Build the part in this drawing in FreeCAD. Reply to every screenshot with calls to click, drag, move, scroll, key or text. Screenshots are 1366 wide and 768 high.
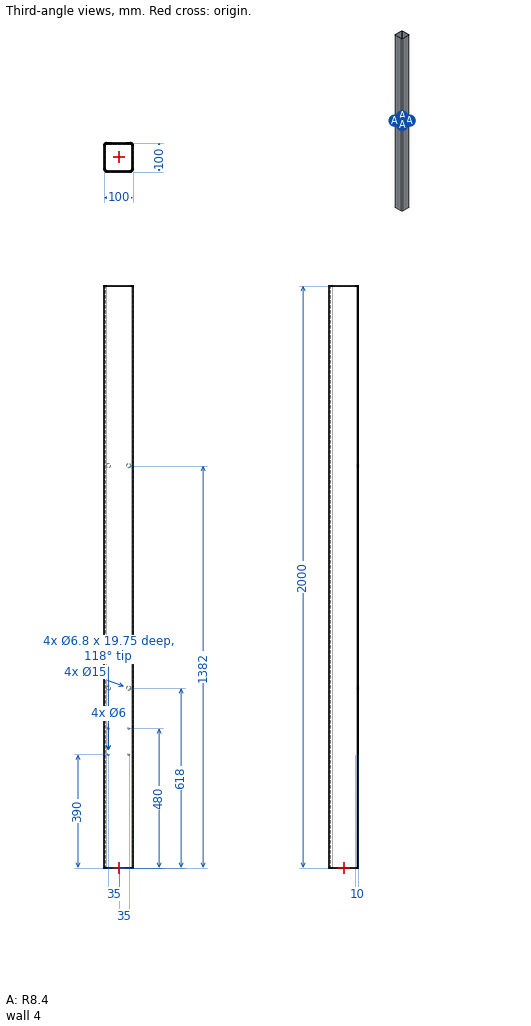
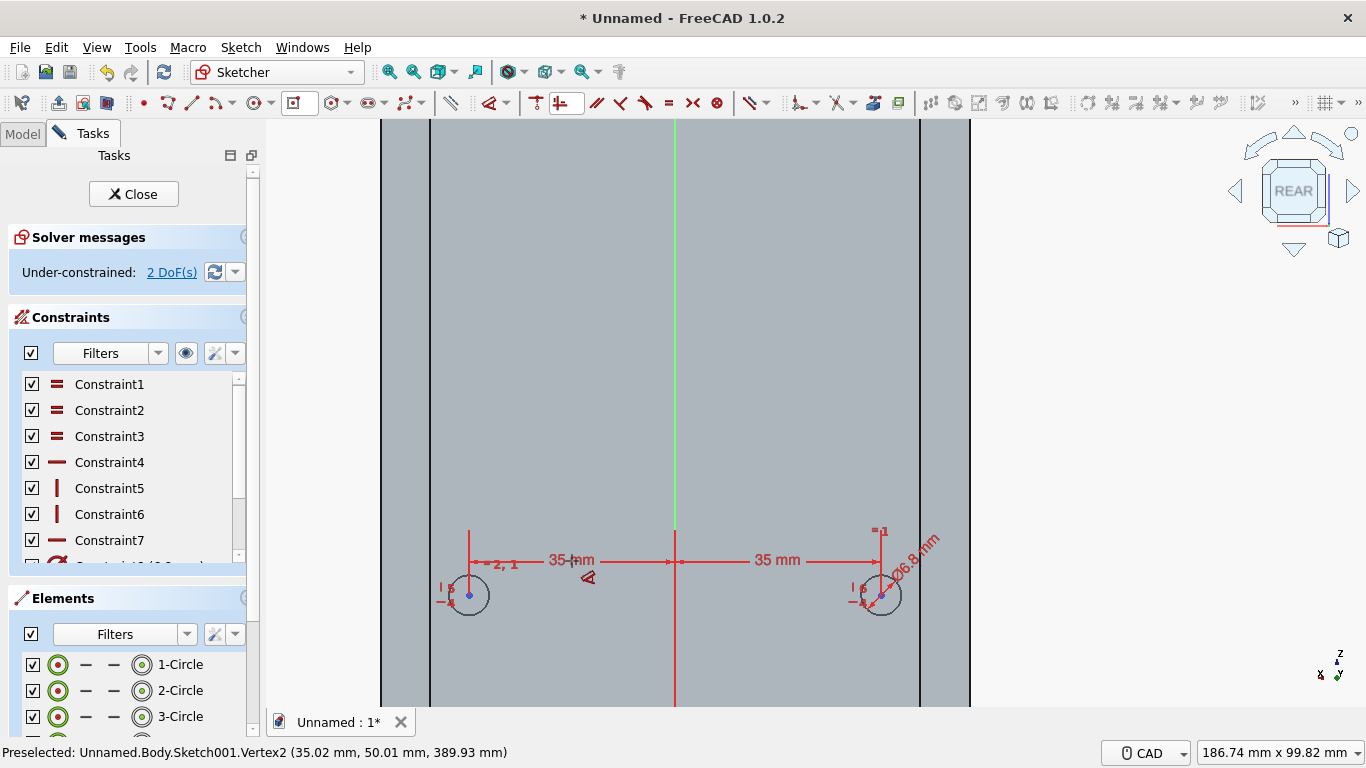
click(881, 595)
click(915, 637)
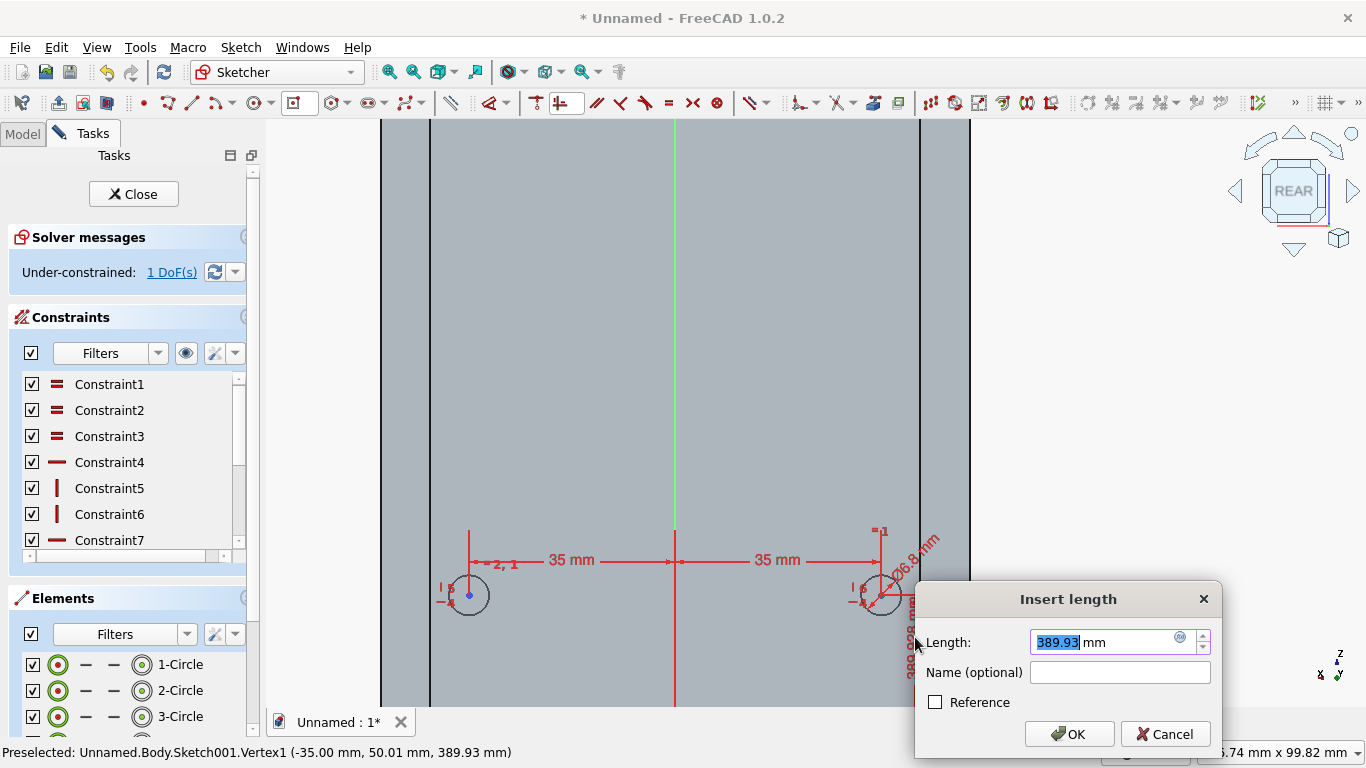
text(390)
key(Return)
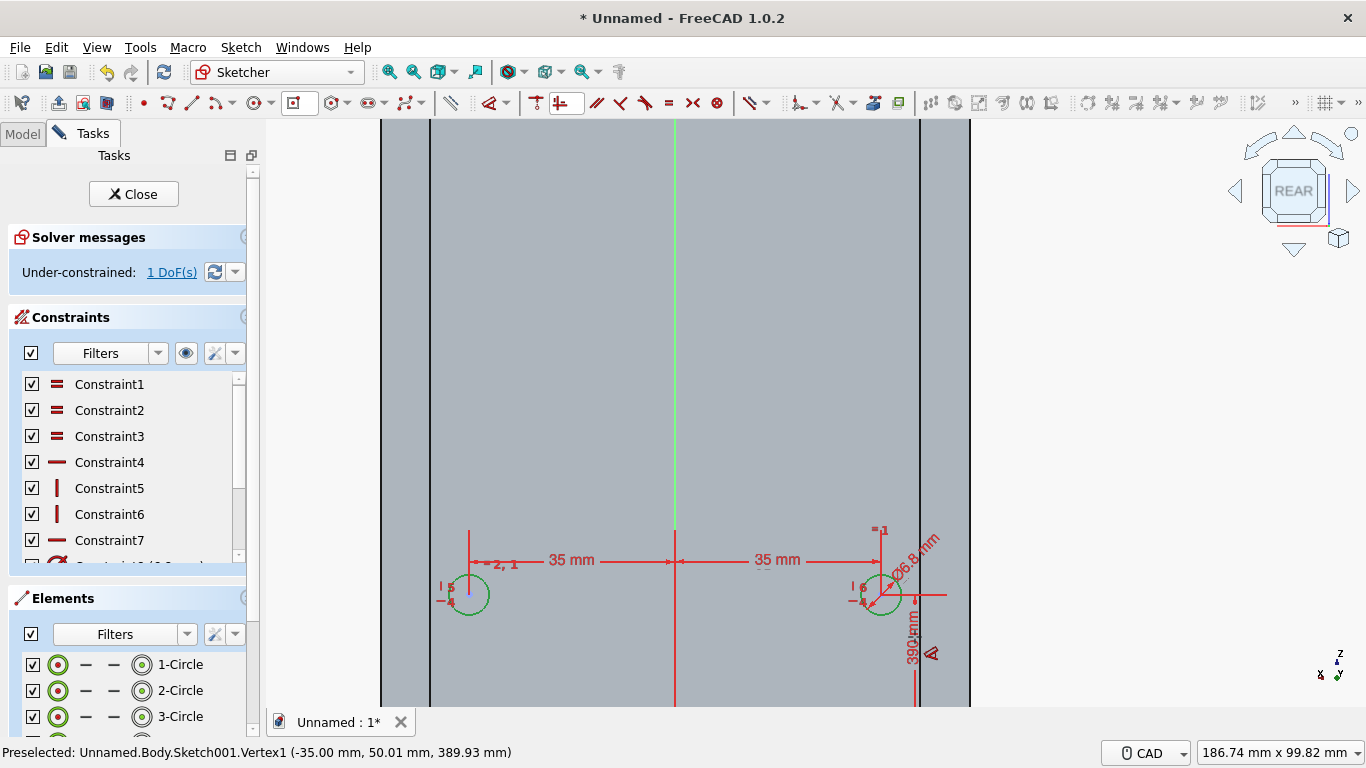
scroll(895, 582, down, 2)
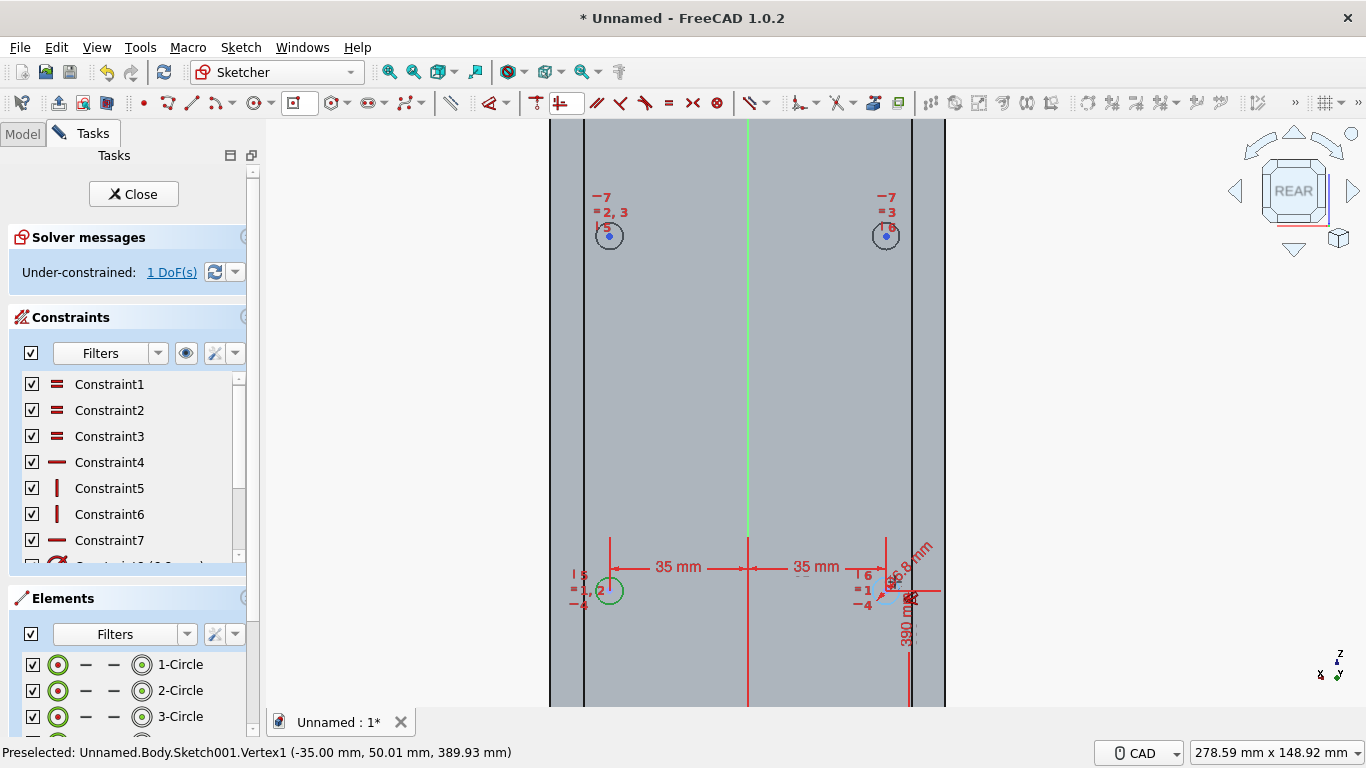
click(610, 236)
click(576, 458)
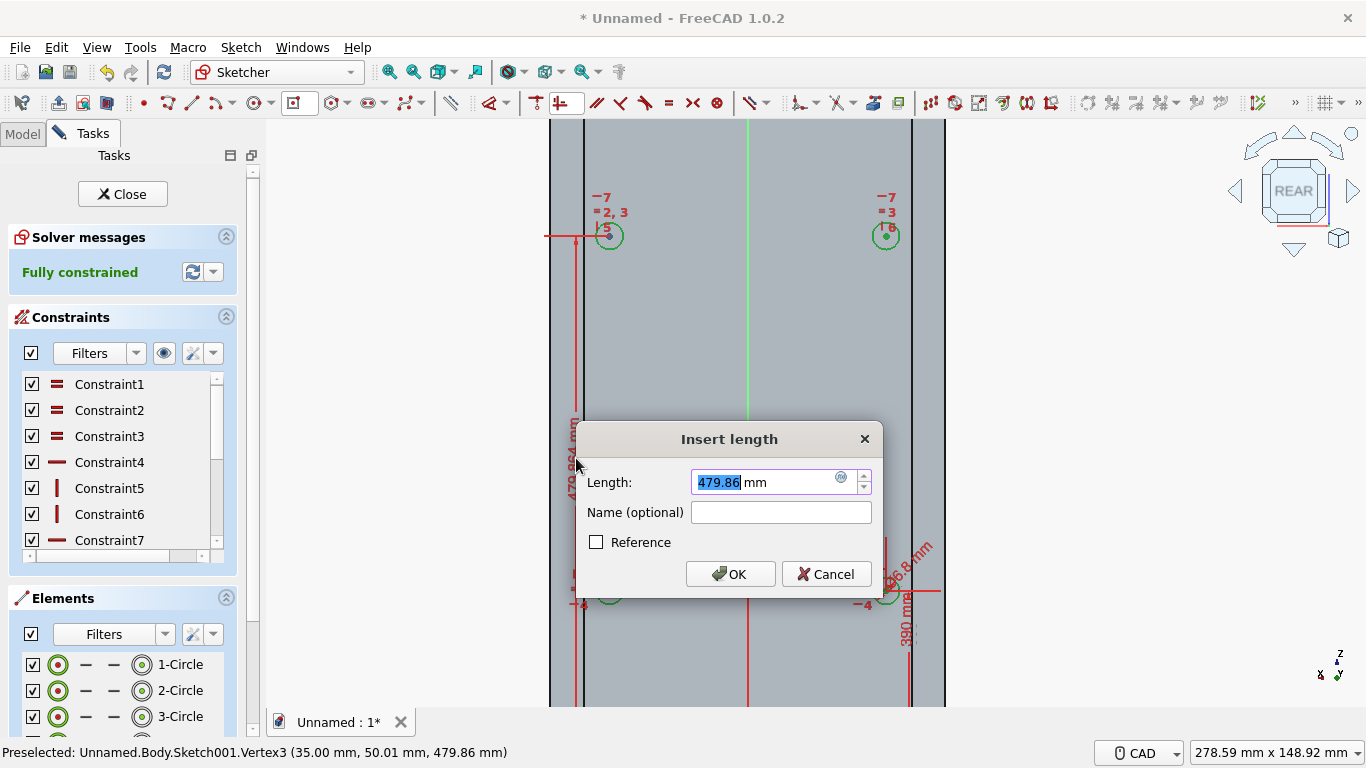
text(480)
key(Return)
key(Escape)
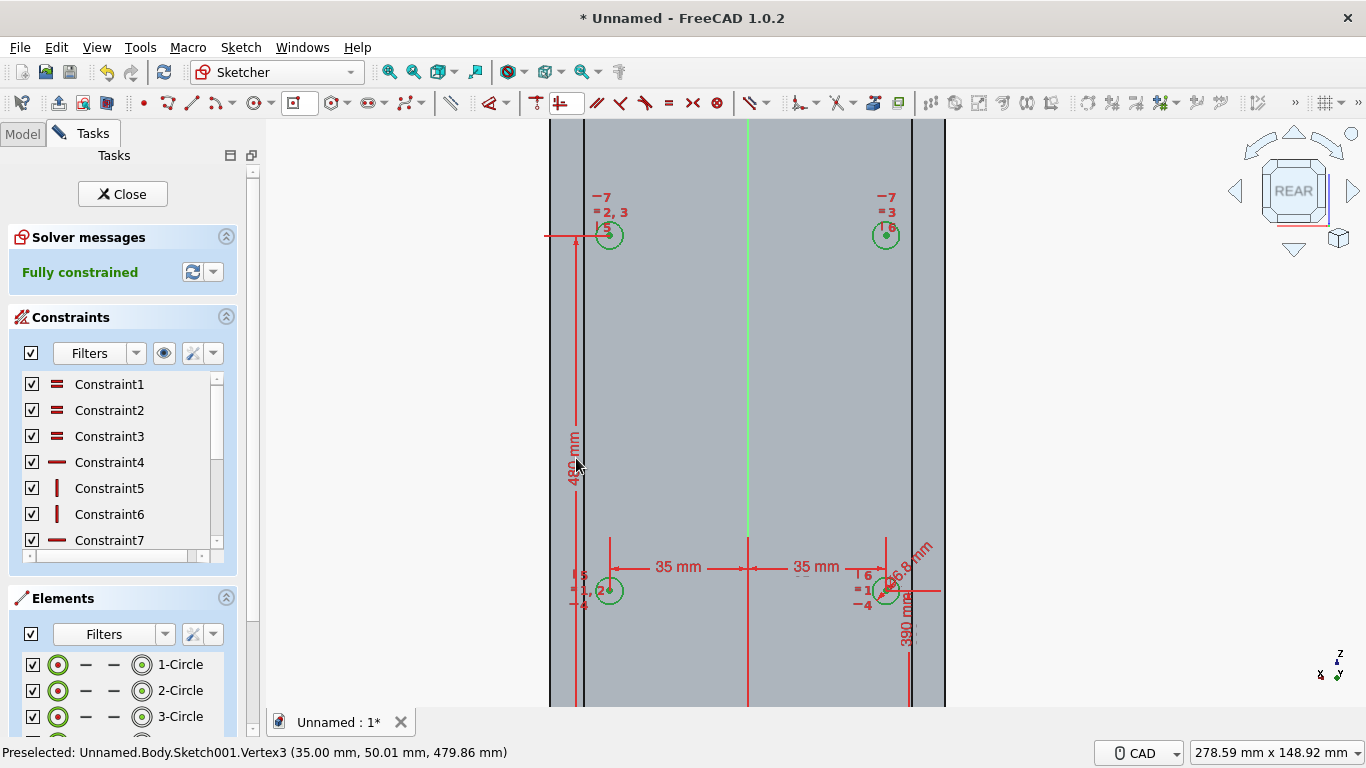
click(123, 194)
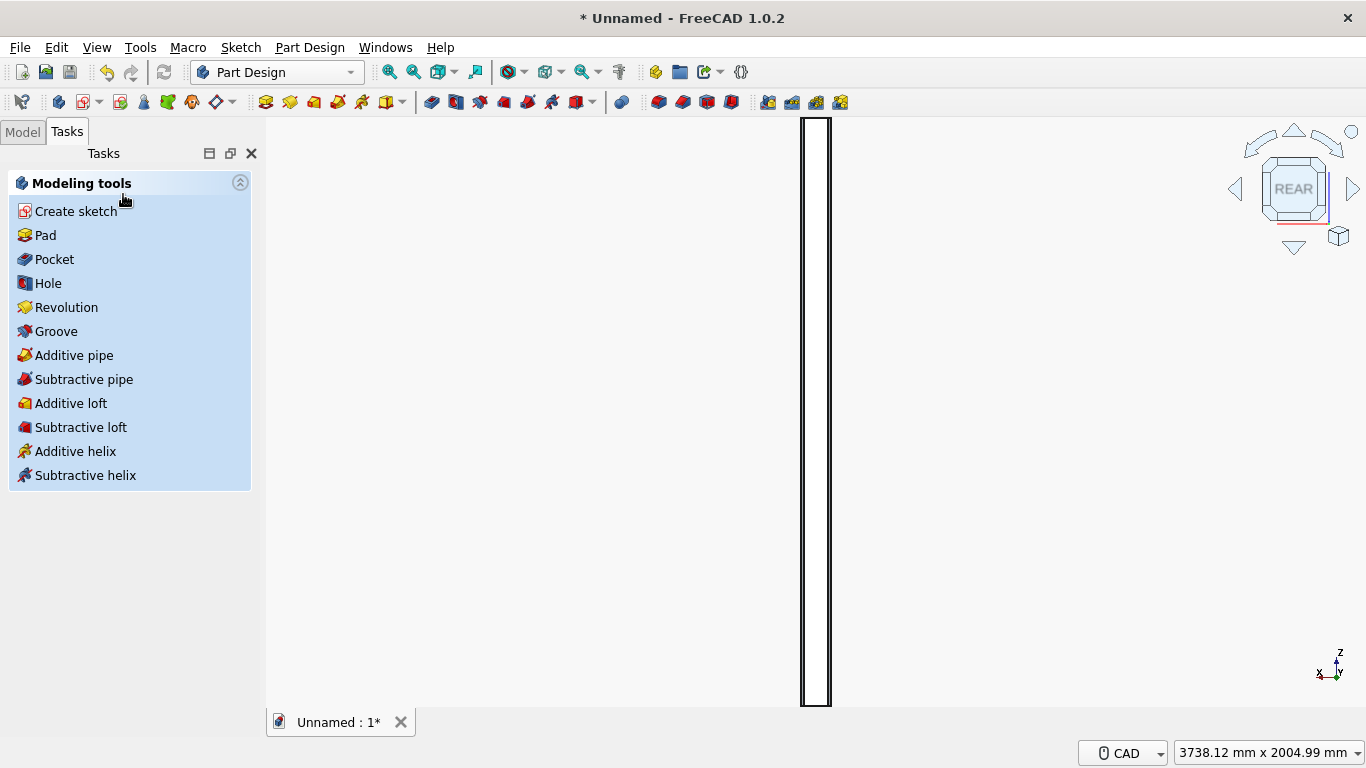
click(456, 102)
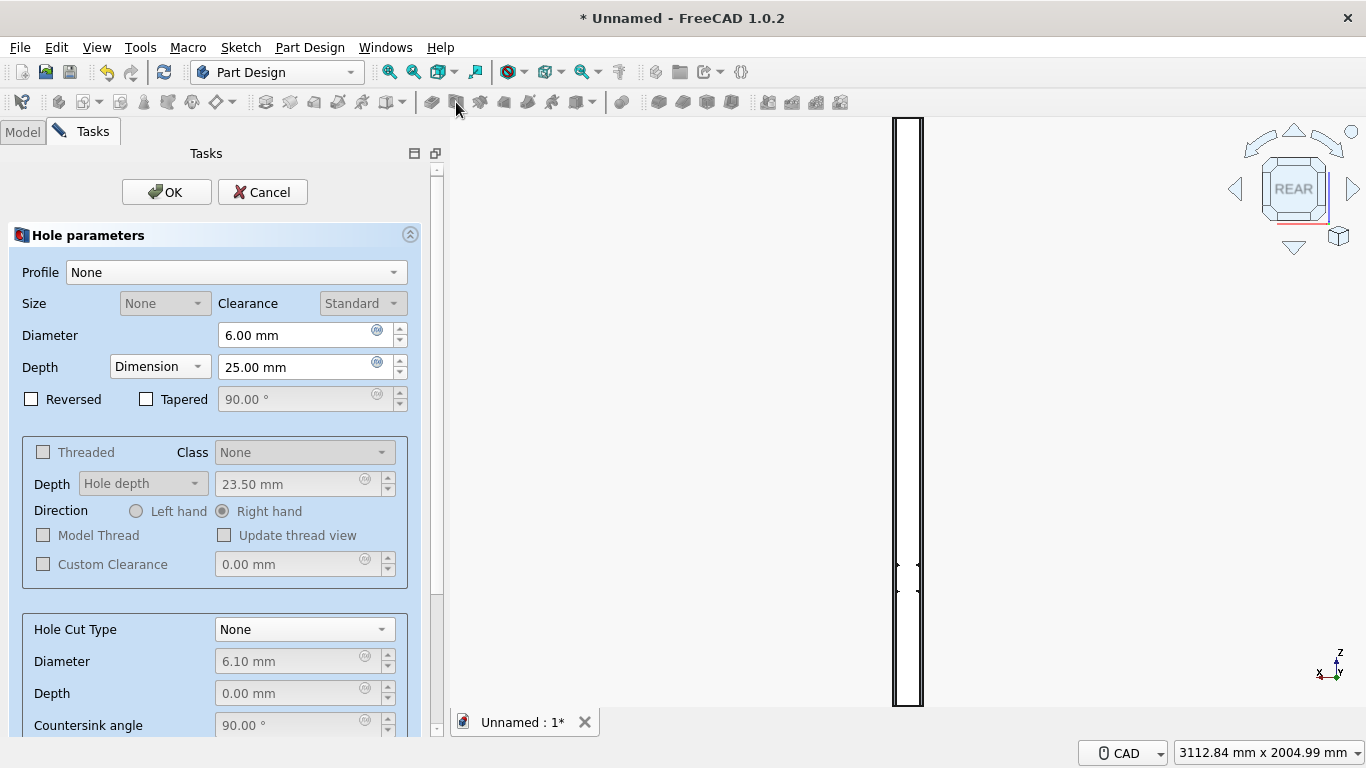
triple_click(305, 335)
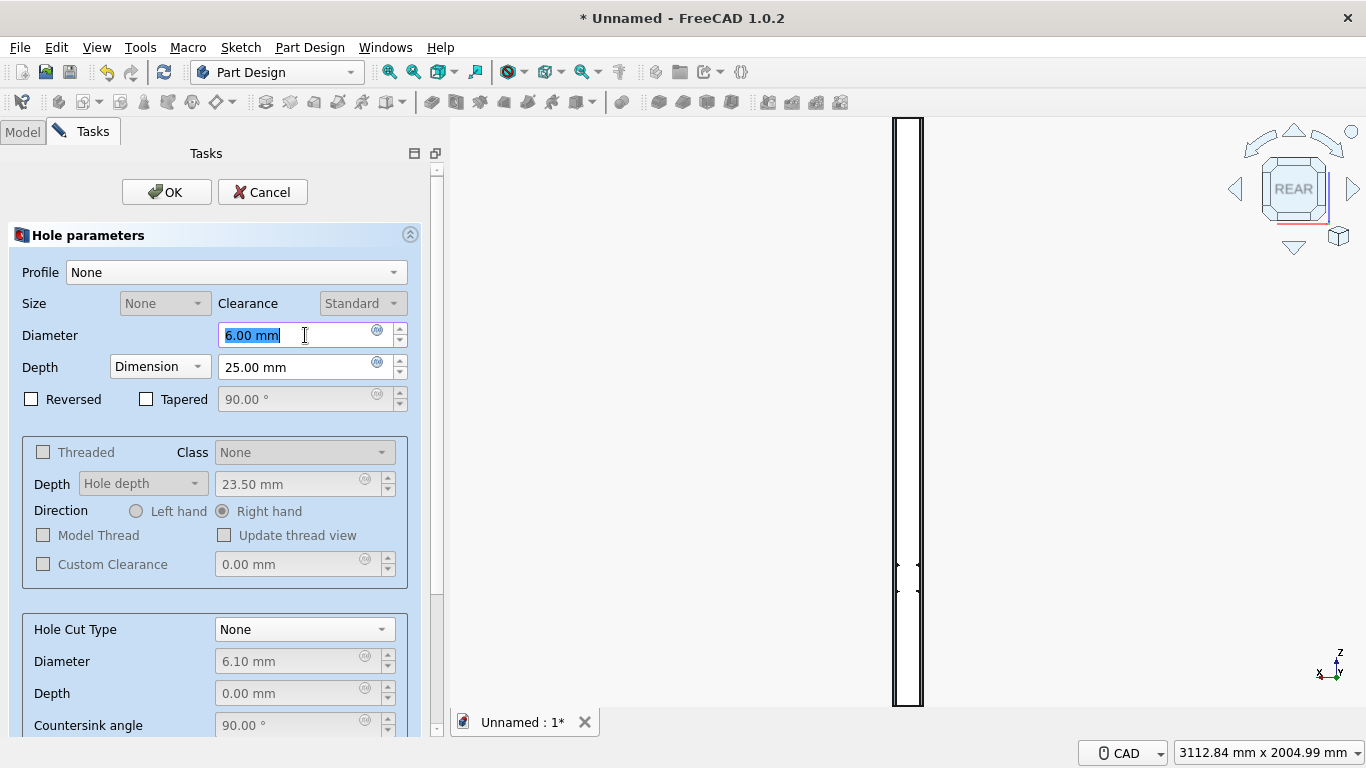
text(6.8)
key(Tab)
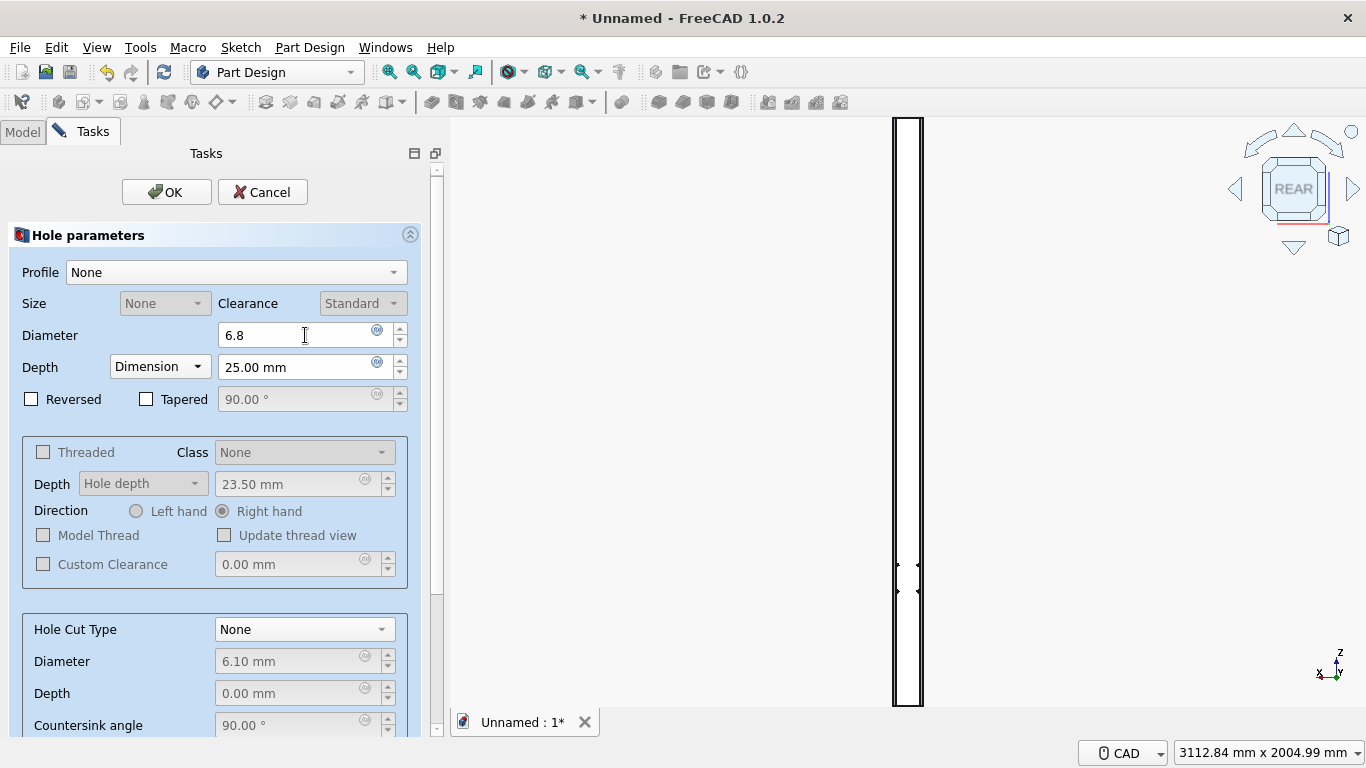
triple_click(305, 367)